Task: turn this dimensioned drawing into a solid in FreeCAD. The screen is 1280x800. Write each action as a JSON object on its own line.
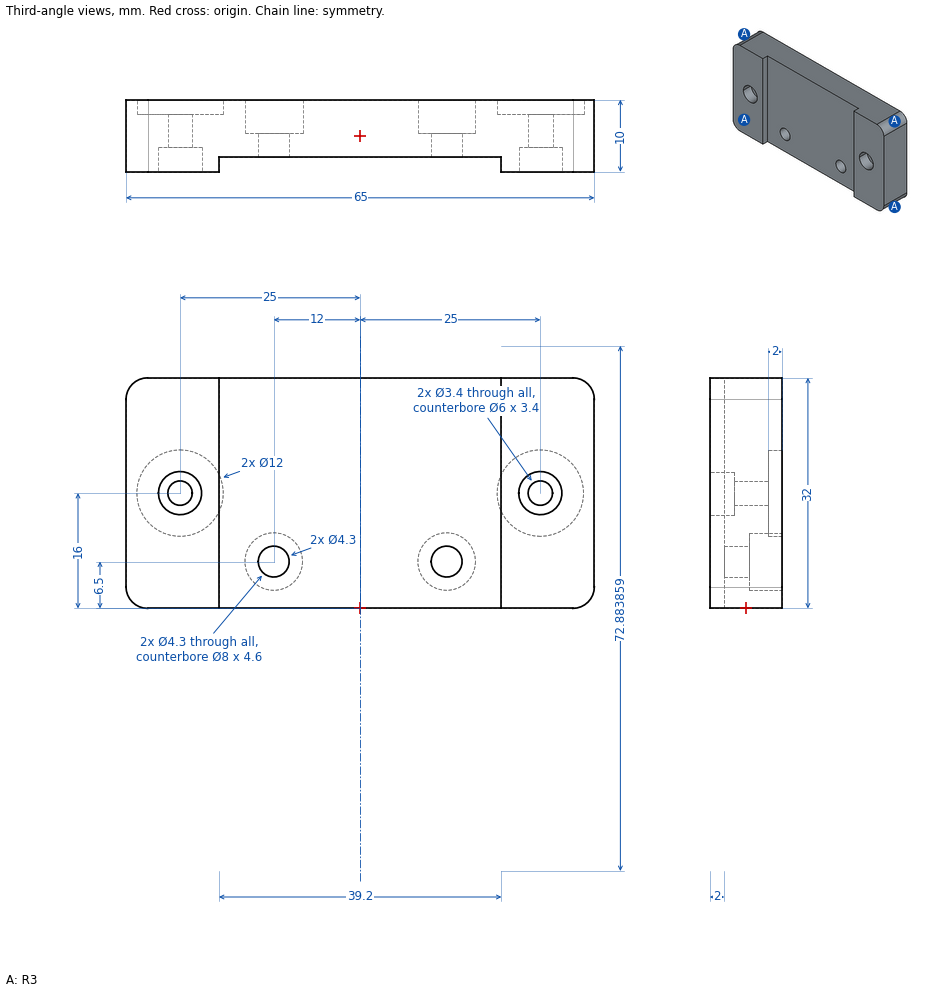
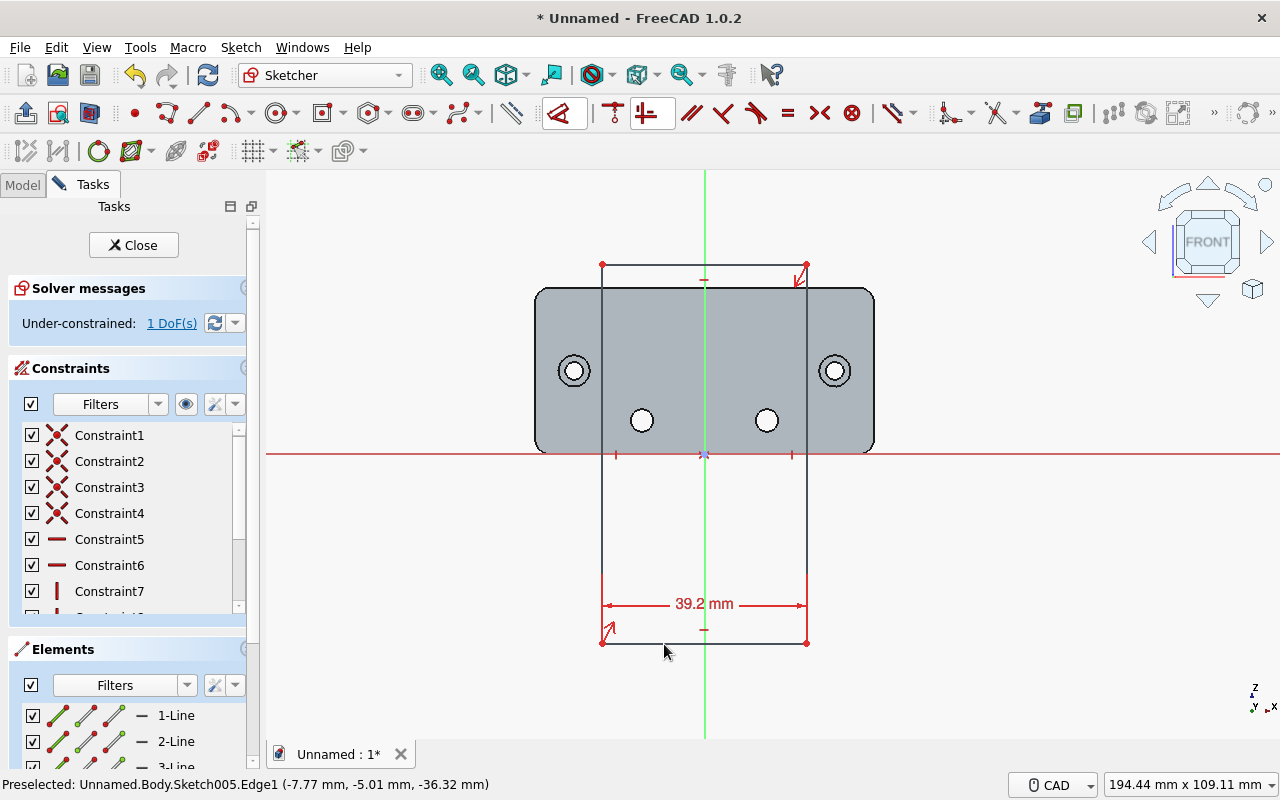
{"action": "left_click", "coordinate": [807, 530]}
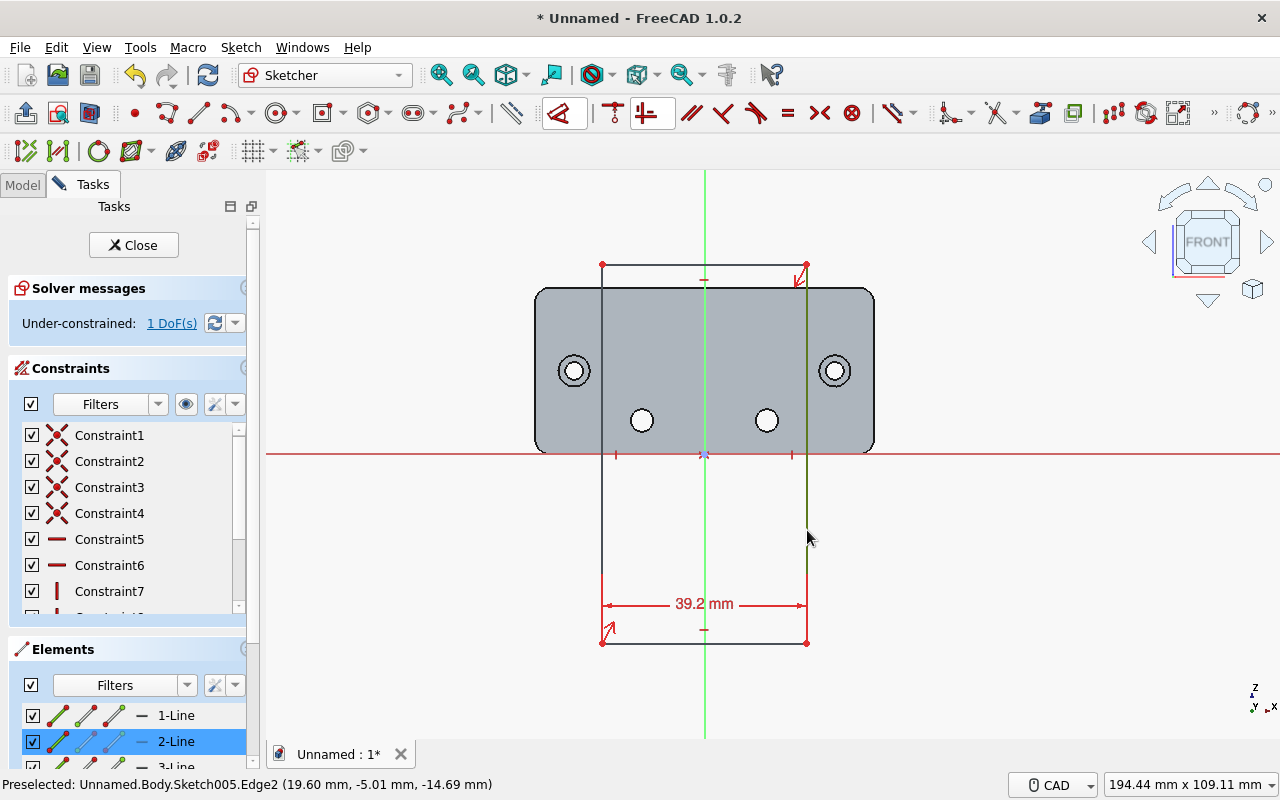
{"action": "key", "text": "i"}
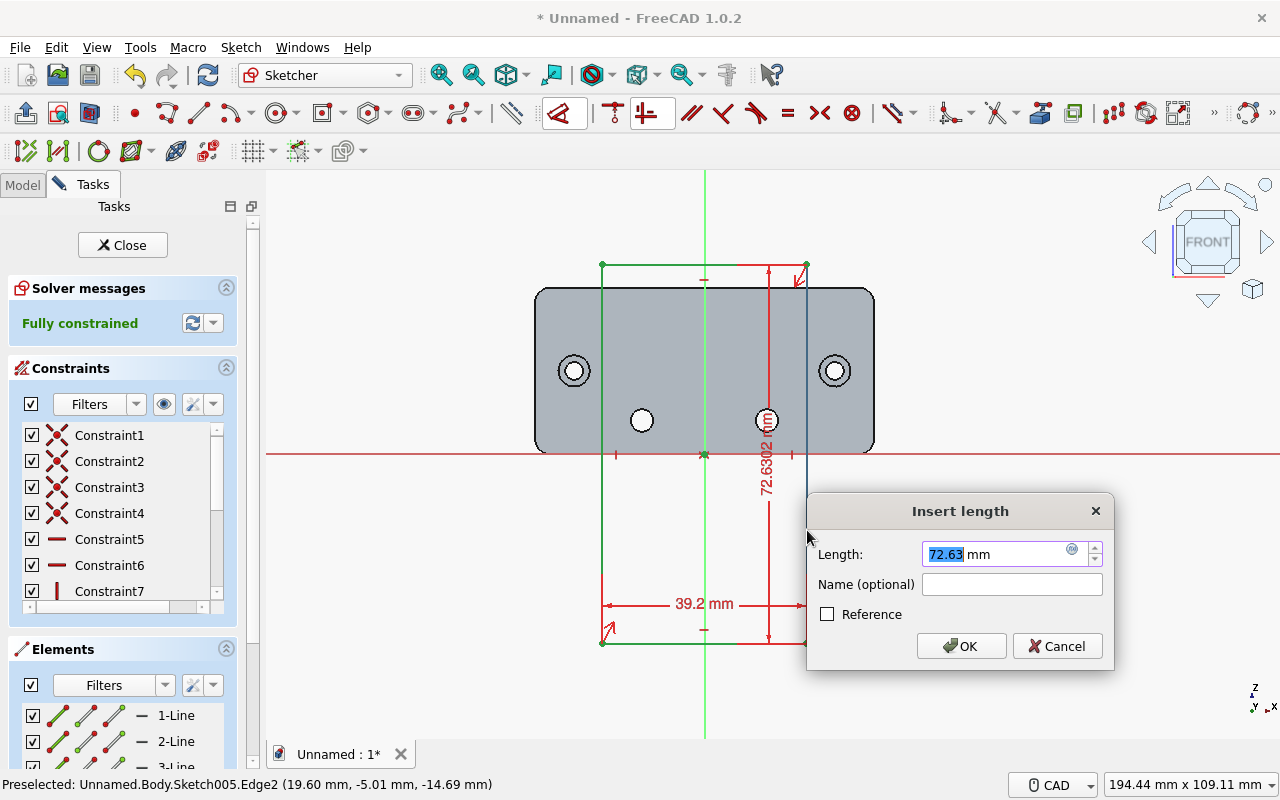
{"action": "type", "text": "72.883859"}
{"action": "key", "text": "Return"}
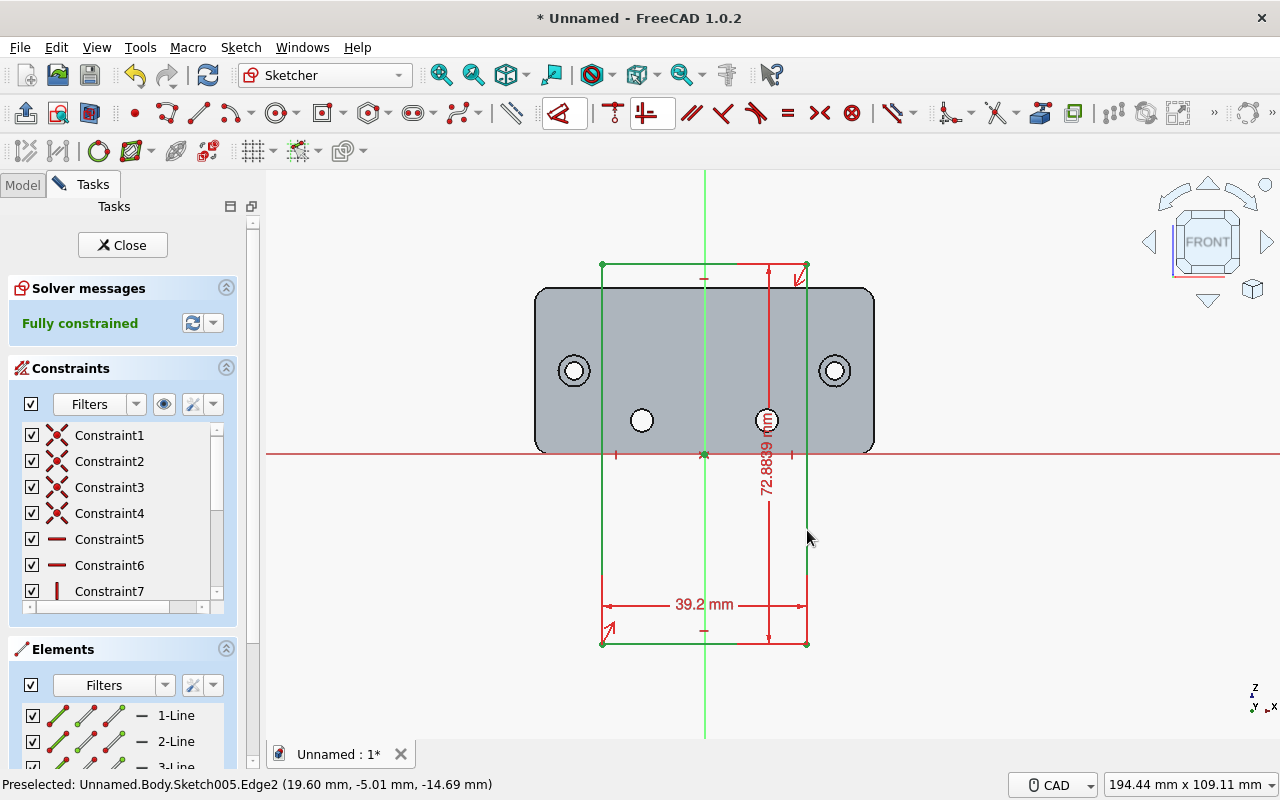
{"action": "left_click", "coordinate": [123, 245]}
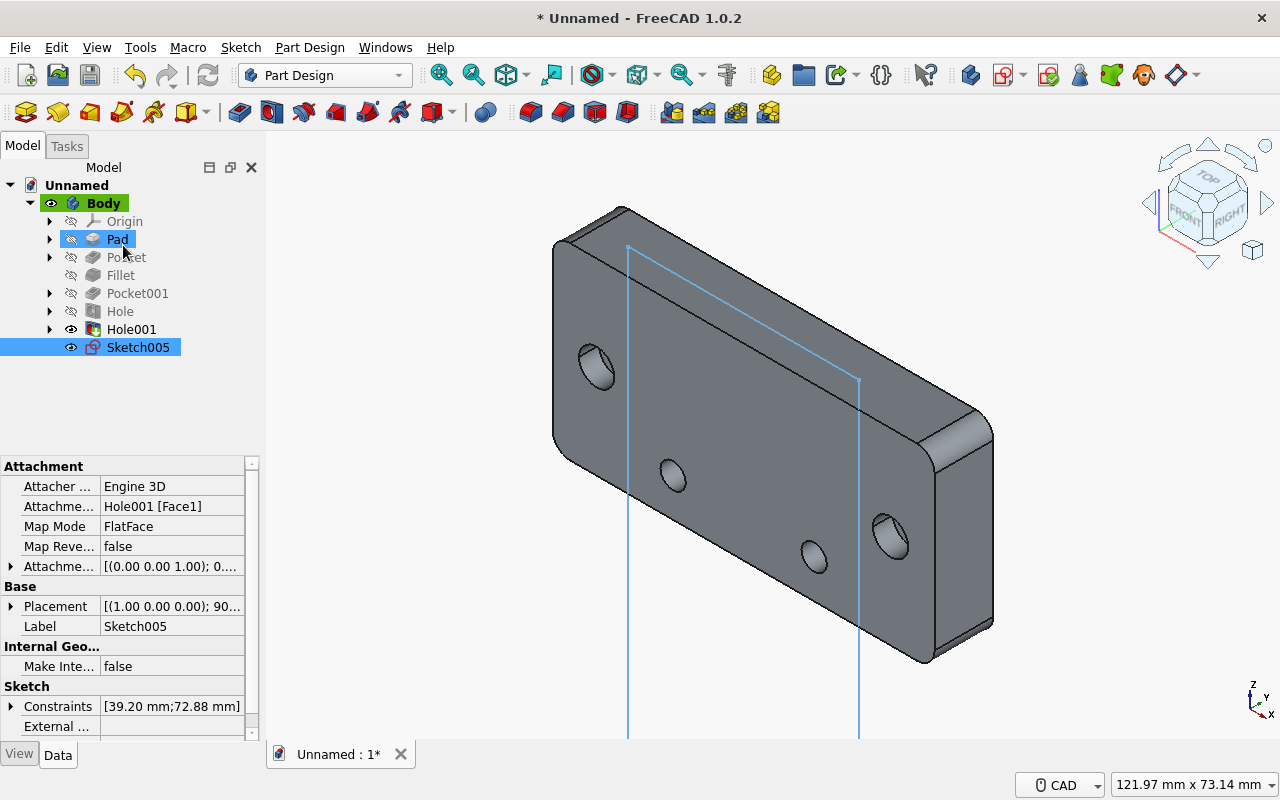
{"action": "left_click", "coordinate": [240, 112]}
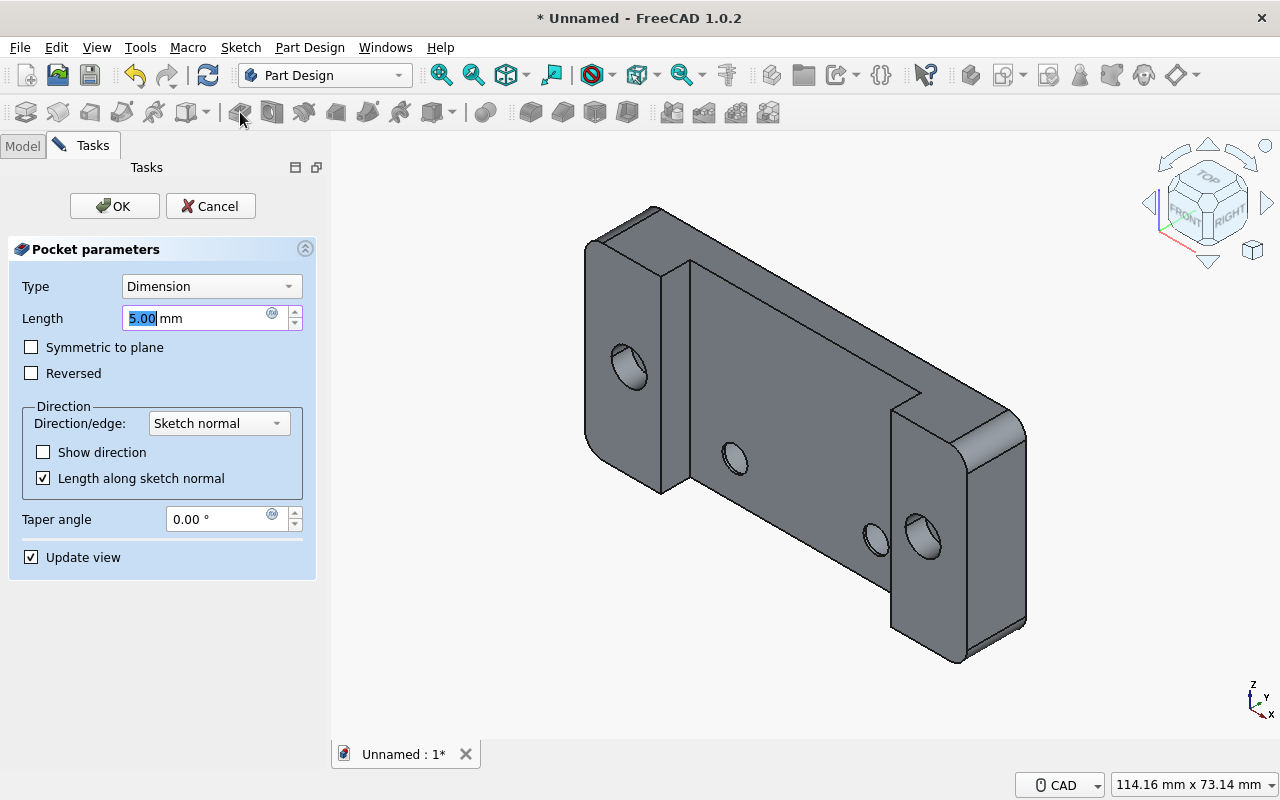
{"action": "type", "text": "2"}
{"action": "key", "text": "Tab"}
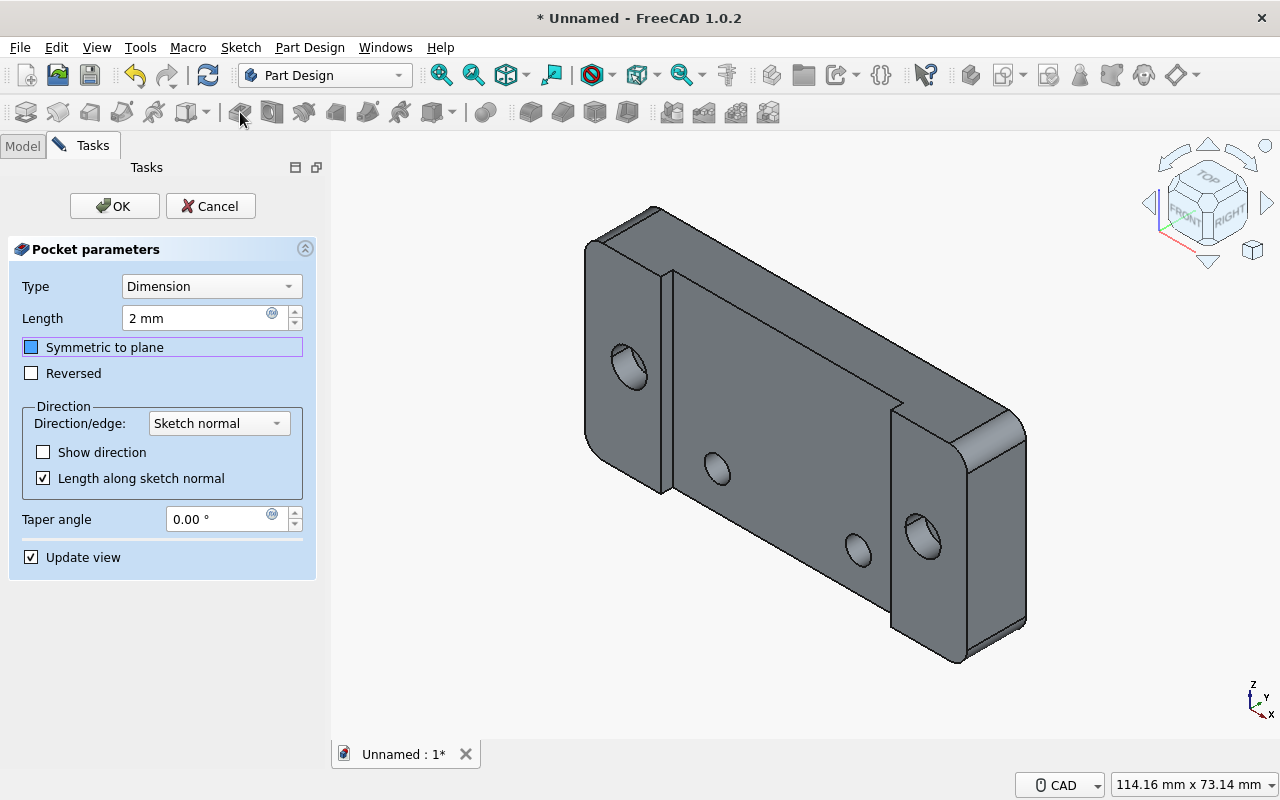
{"action": "left_click", "coordinate": [115, 206]}